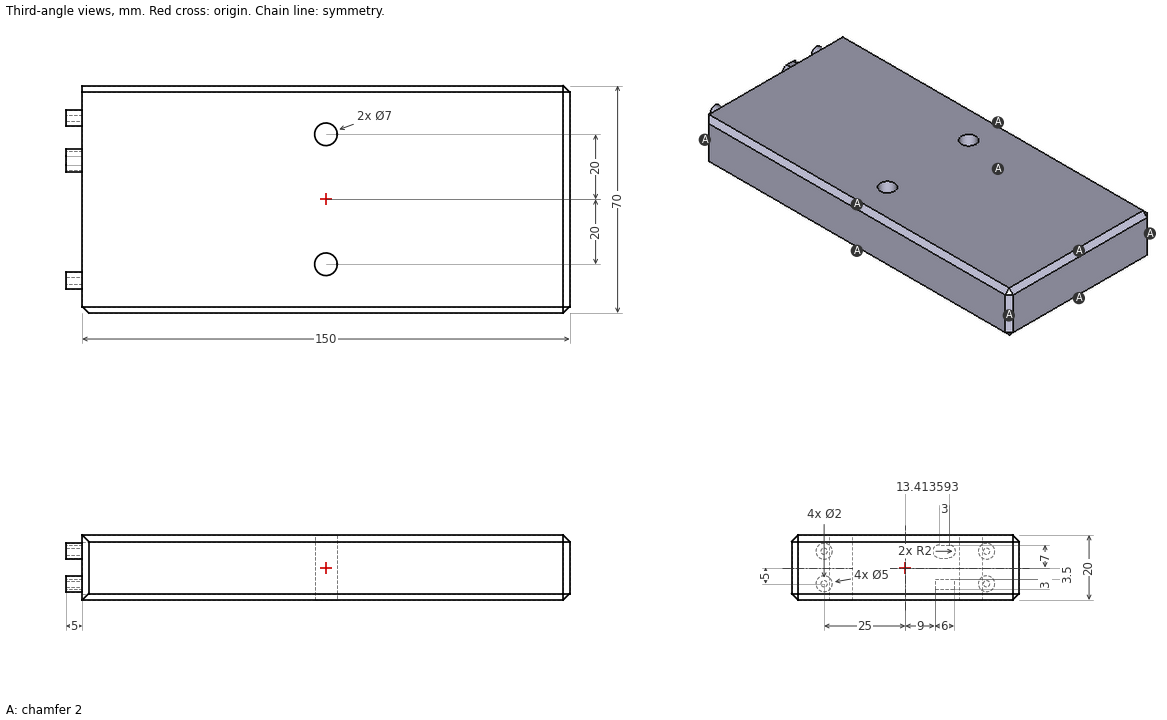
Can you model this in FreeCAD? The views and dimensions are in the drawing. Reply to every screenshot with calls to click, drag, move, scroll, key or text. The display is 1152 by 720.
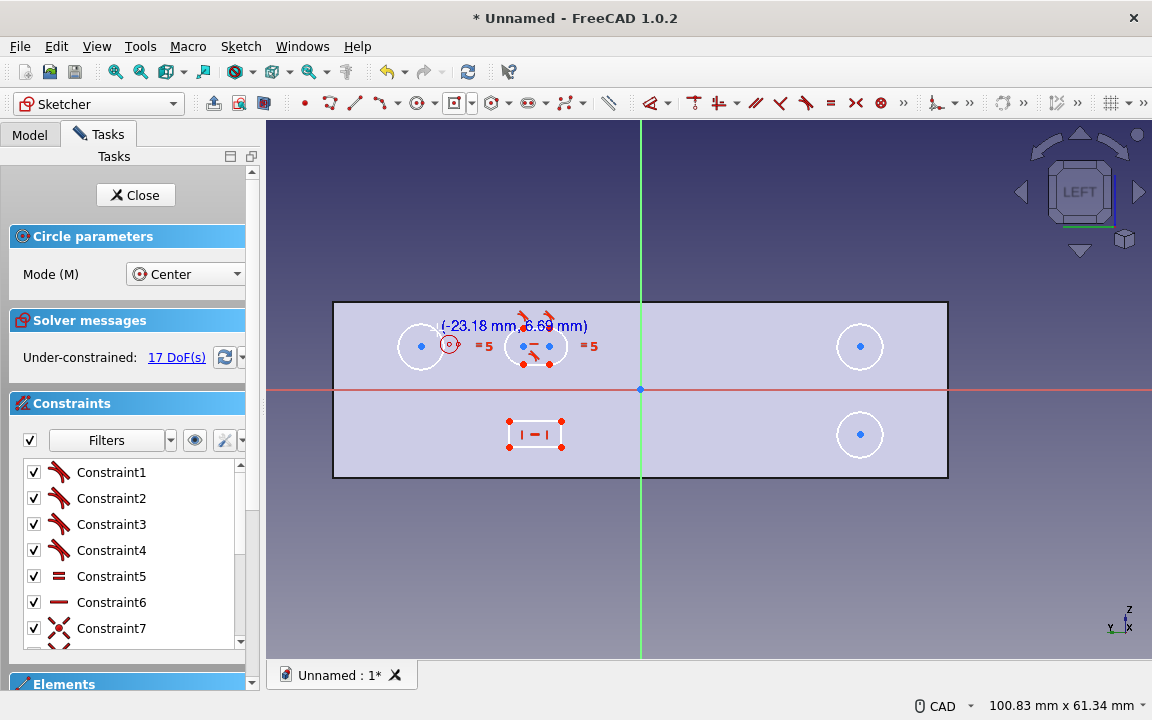
click(421, 434)
click(437, 418)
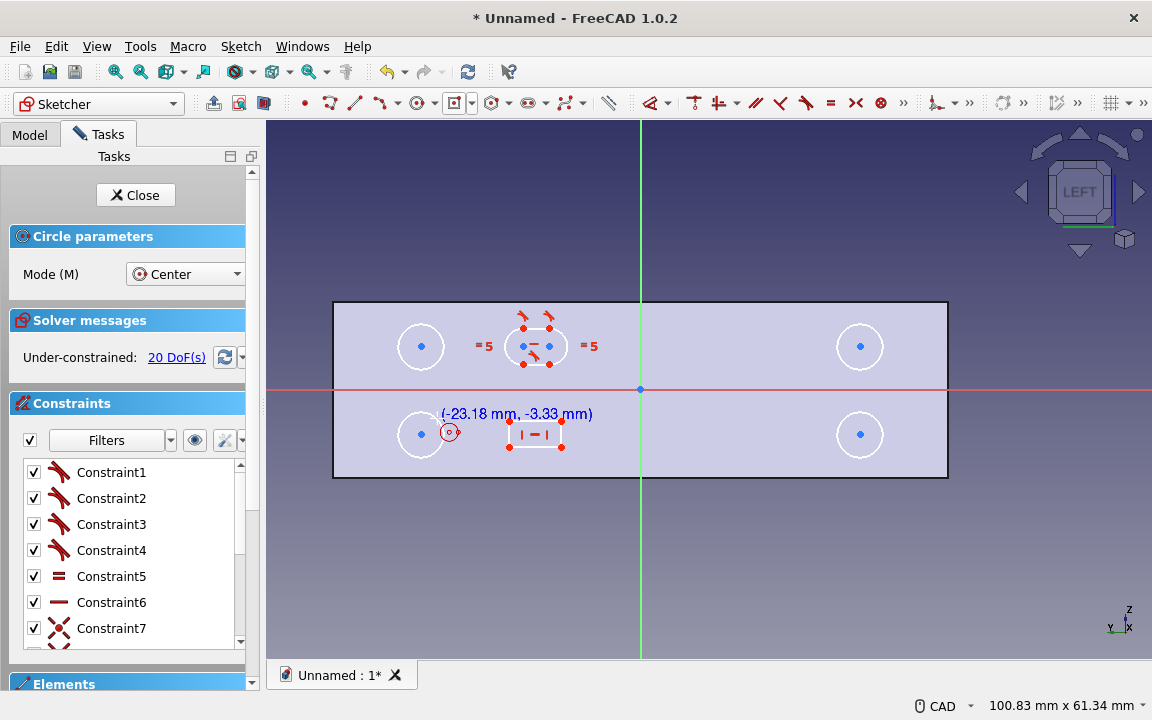
scroll(860, 434, up, 5)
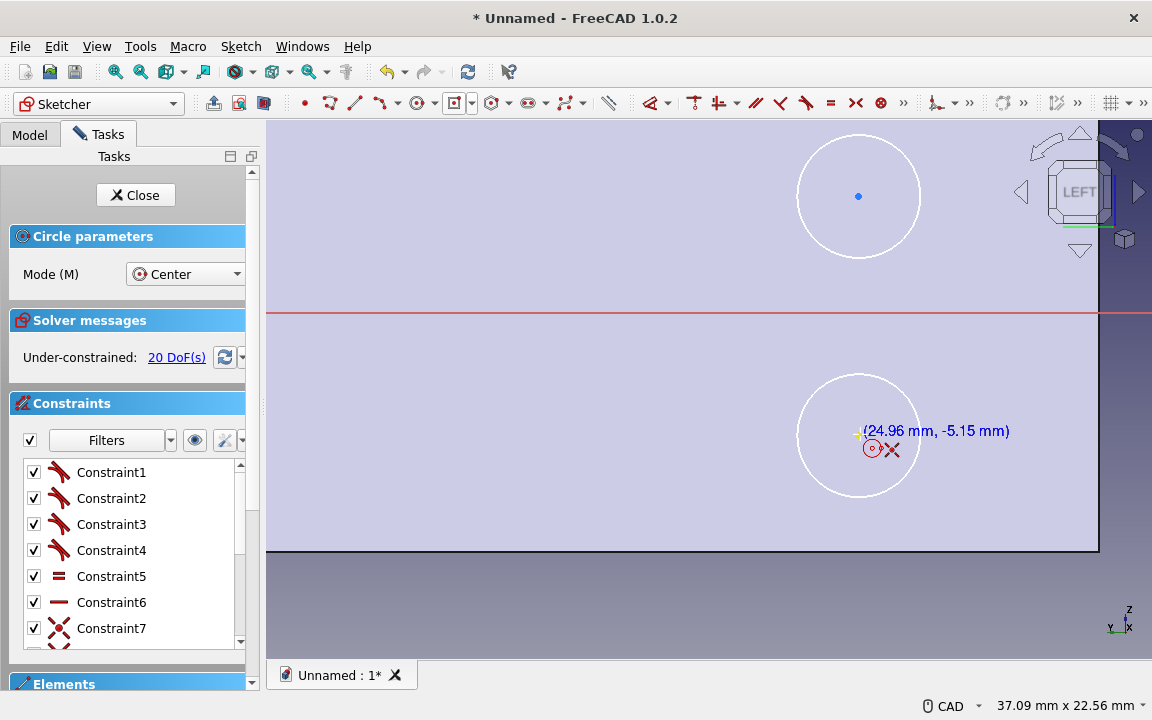
click(859, 436)
click(877, 415)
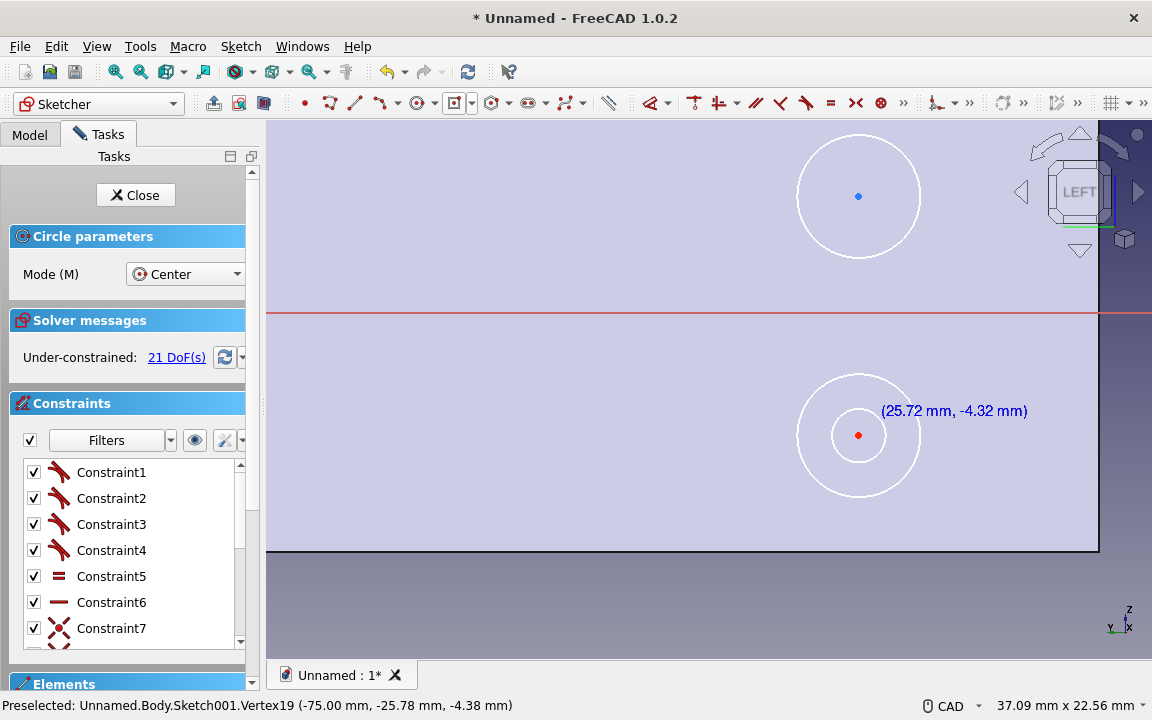
click(859, 197)
click(877, 176)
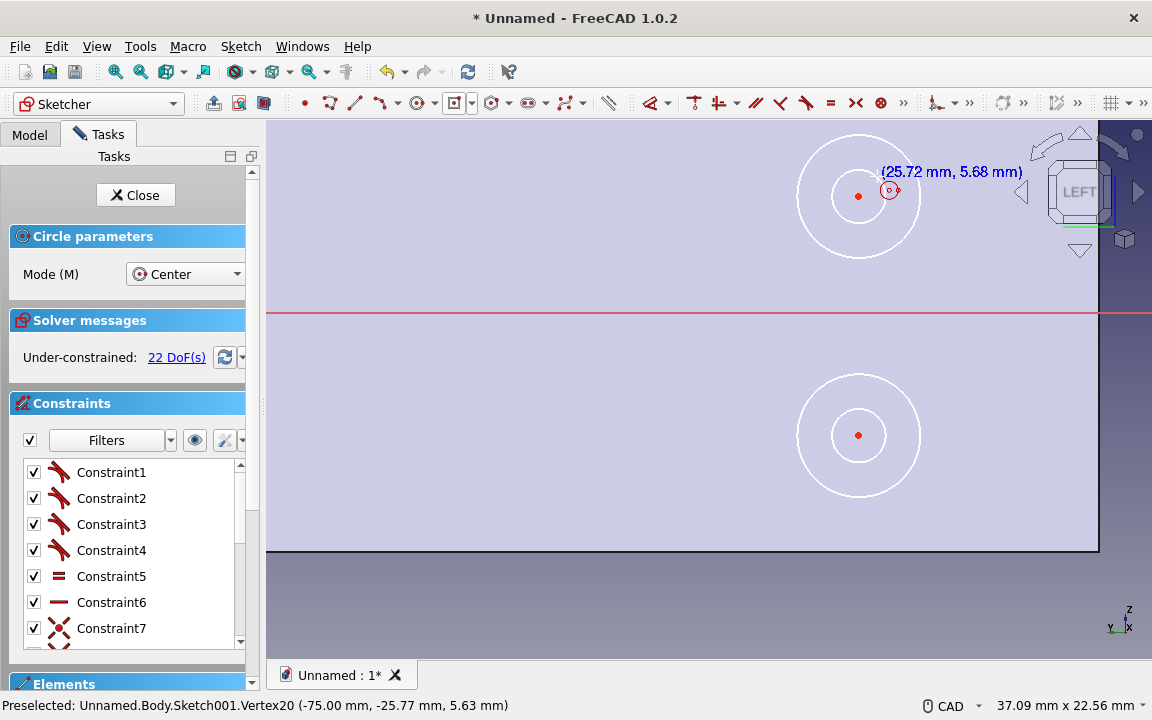
scroll(860, 434, down, 5)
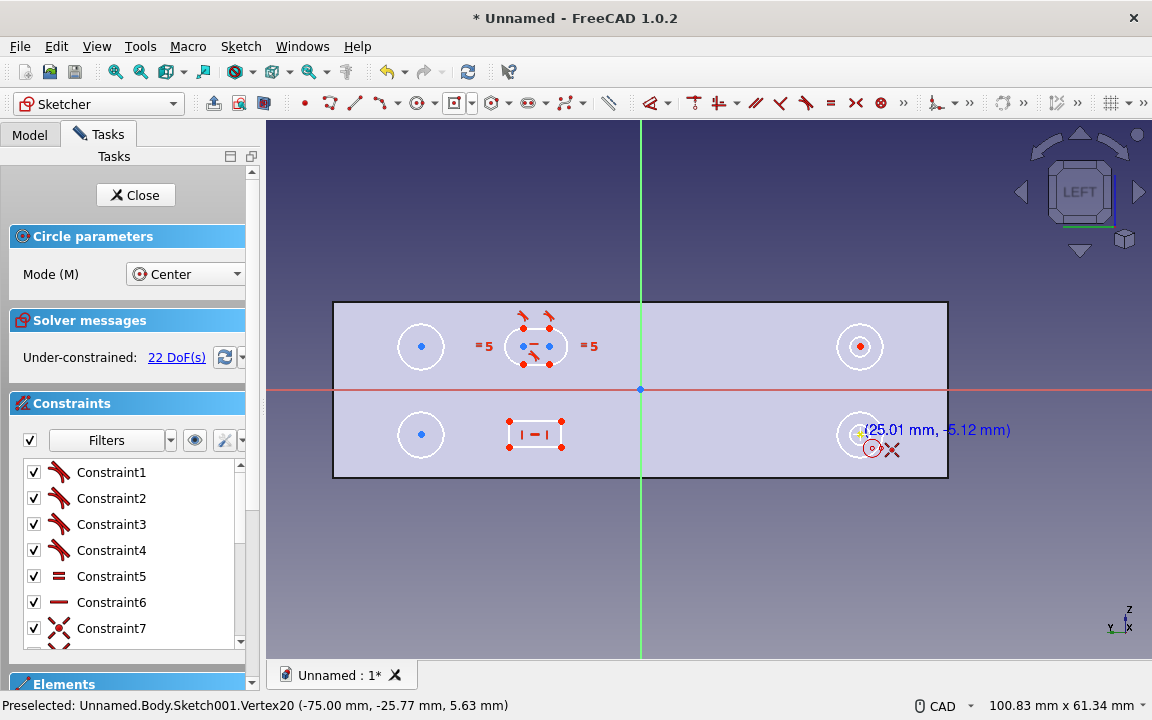
scroll(421, 346, up, 5)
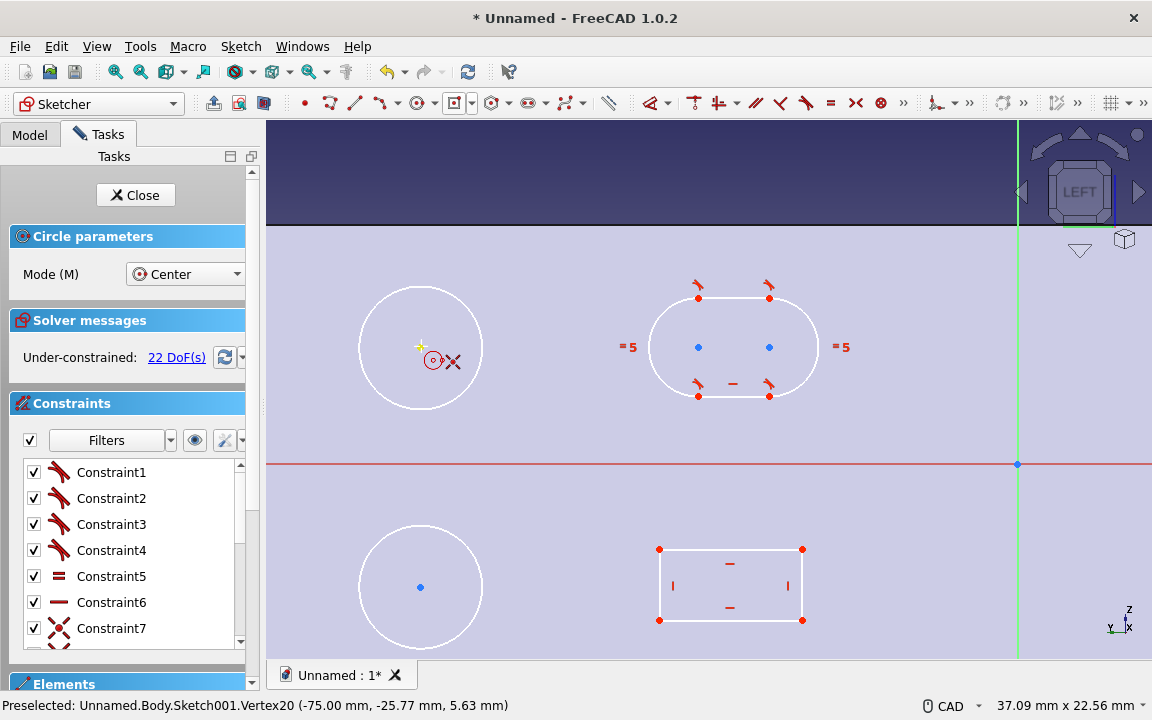
click(421, 348)
click(437, 328)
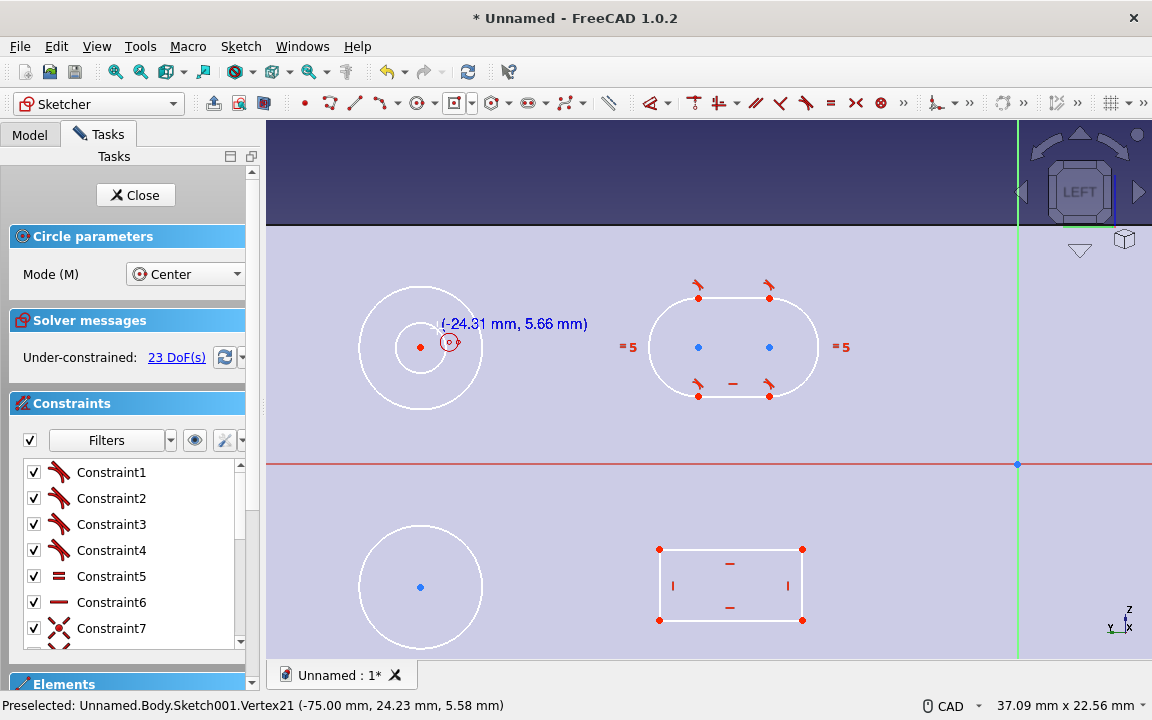
click(421, 587)
click(437, 567)
key(Escape)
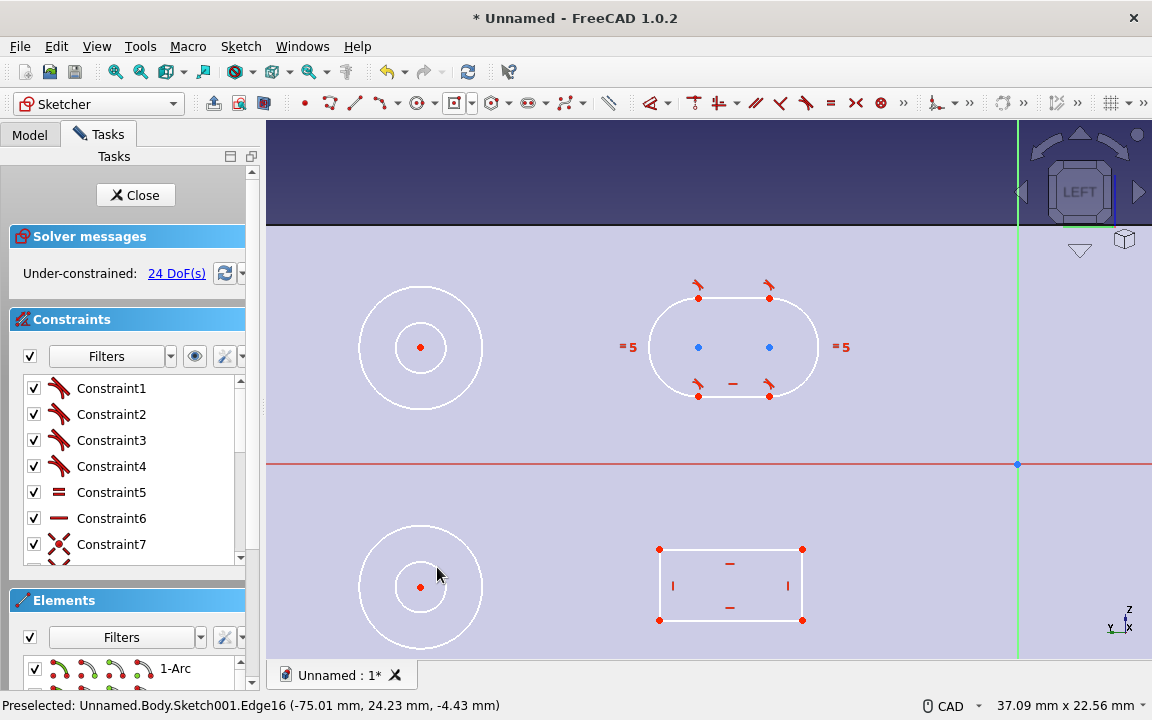
scroll(421, 346, down, 5)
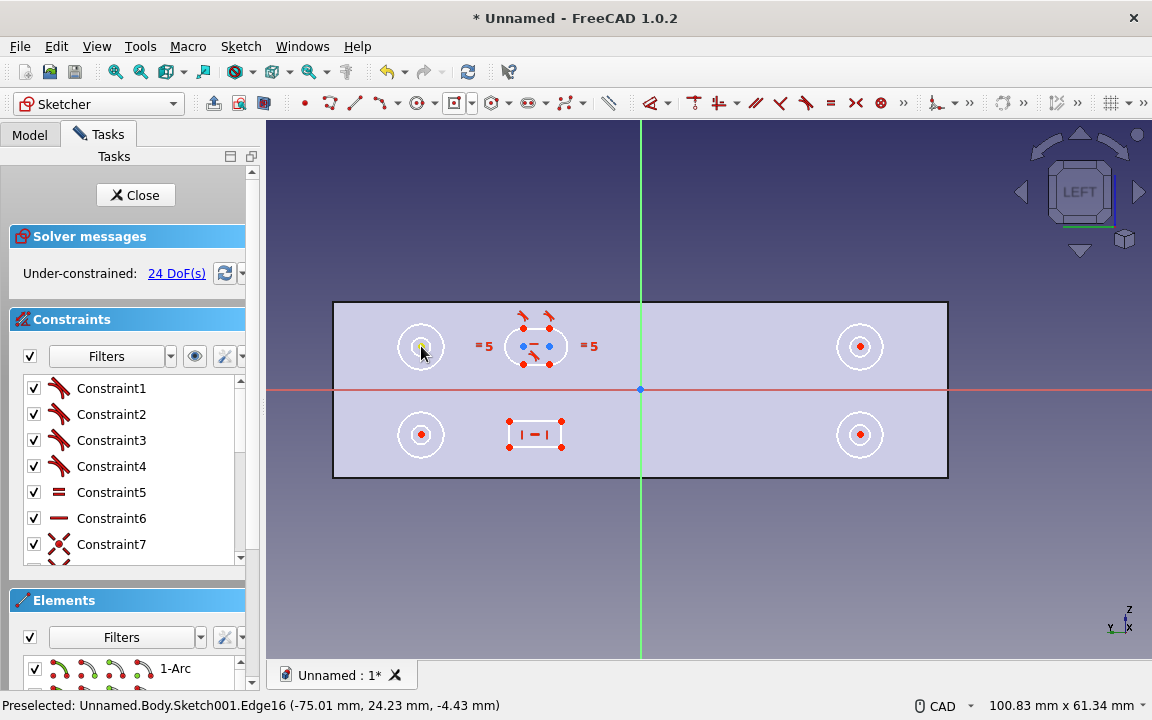
click(876, 419)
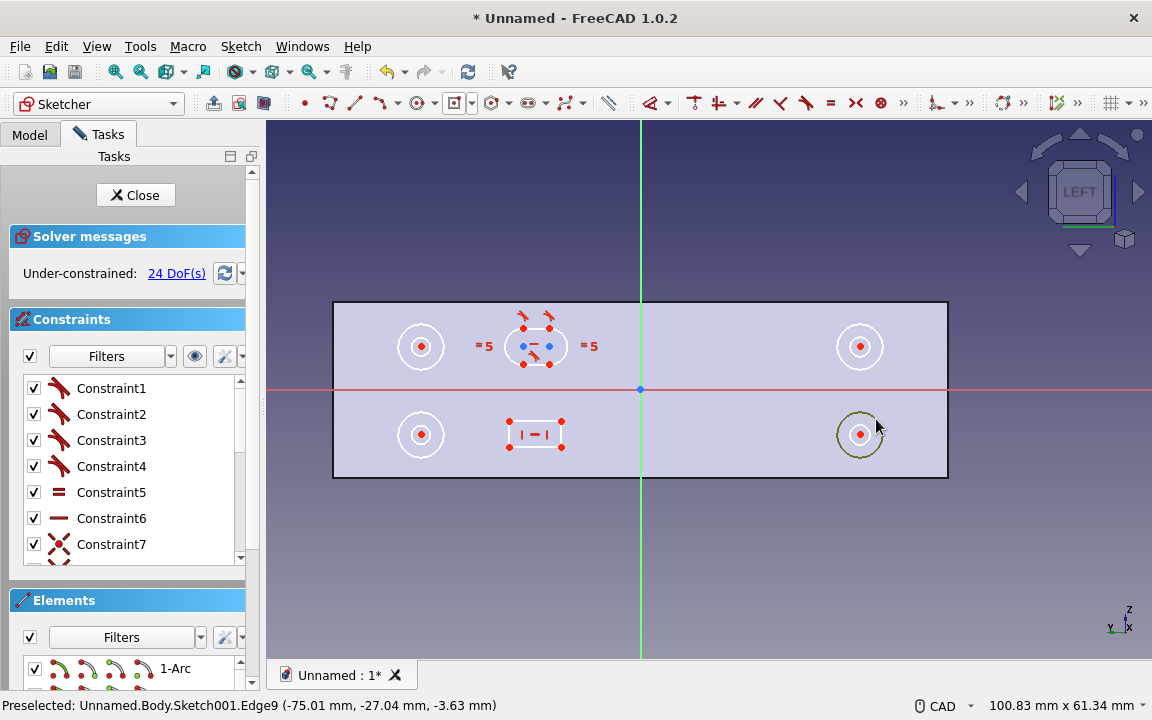
click(876, 331)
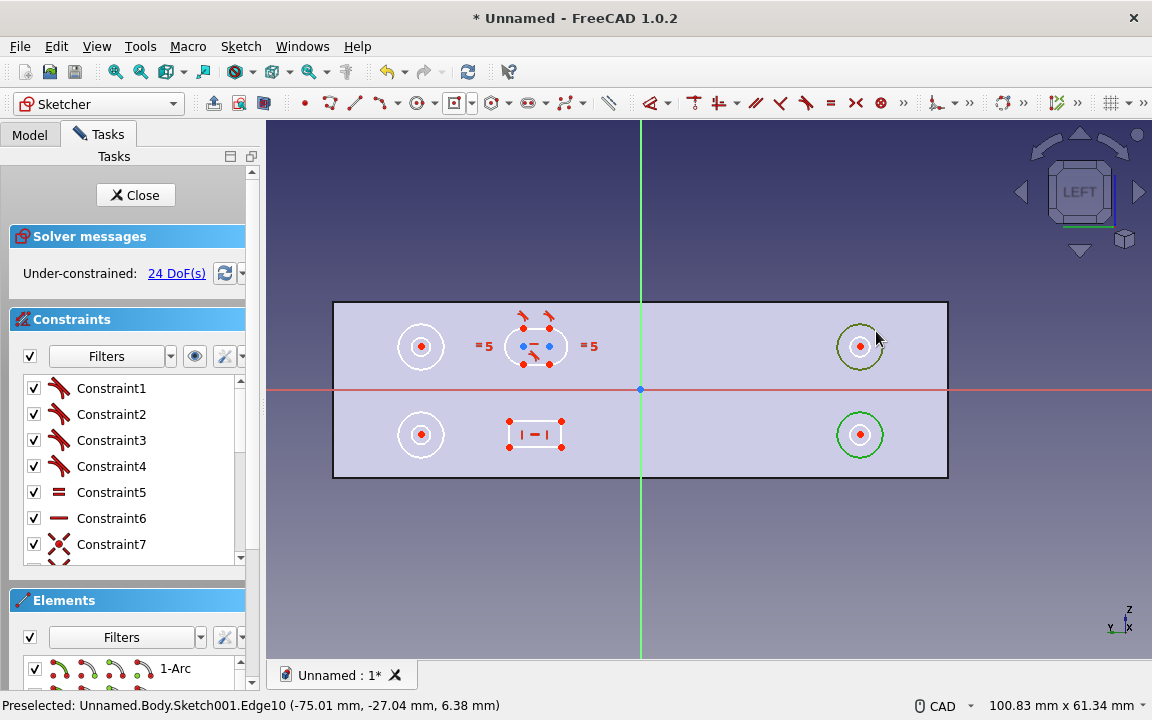
click(437, 331)